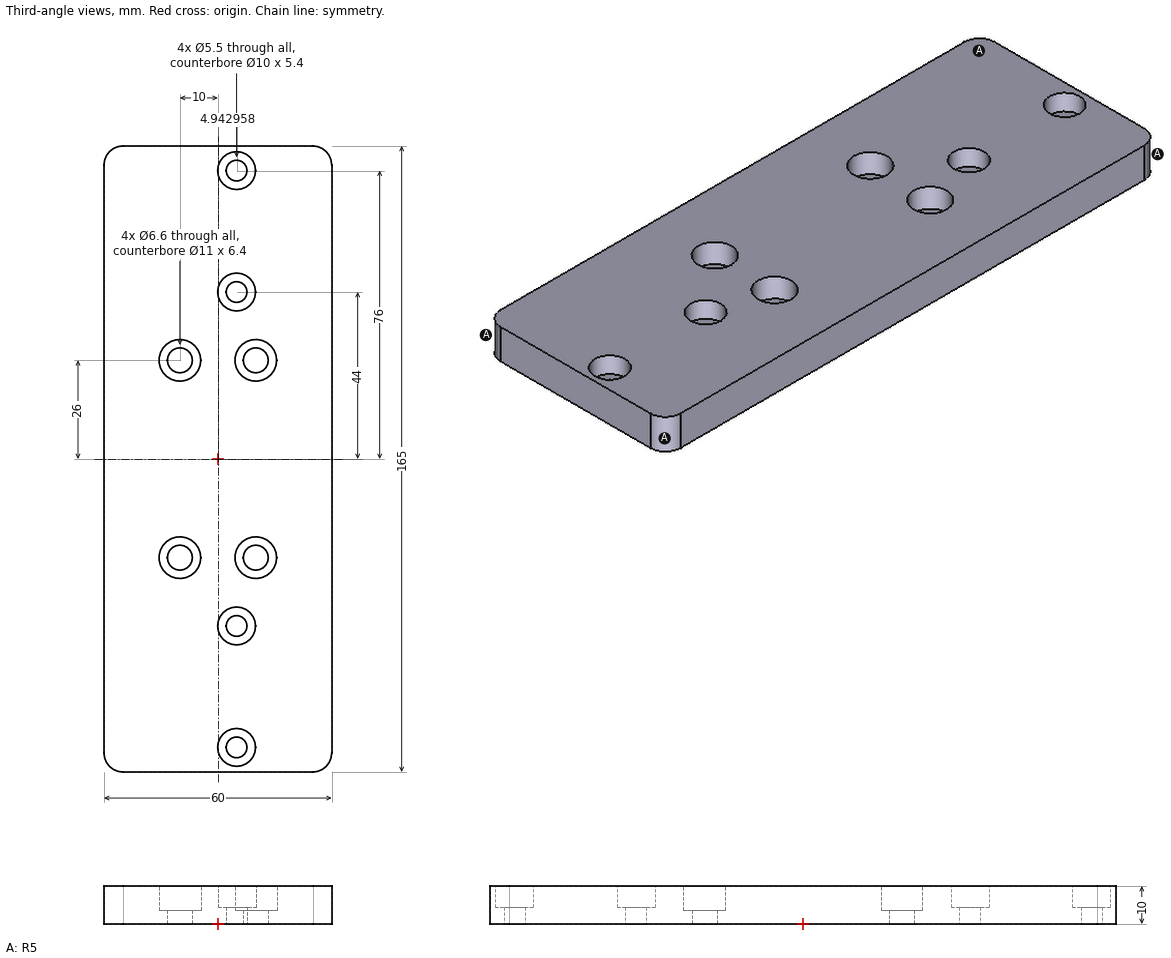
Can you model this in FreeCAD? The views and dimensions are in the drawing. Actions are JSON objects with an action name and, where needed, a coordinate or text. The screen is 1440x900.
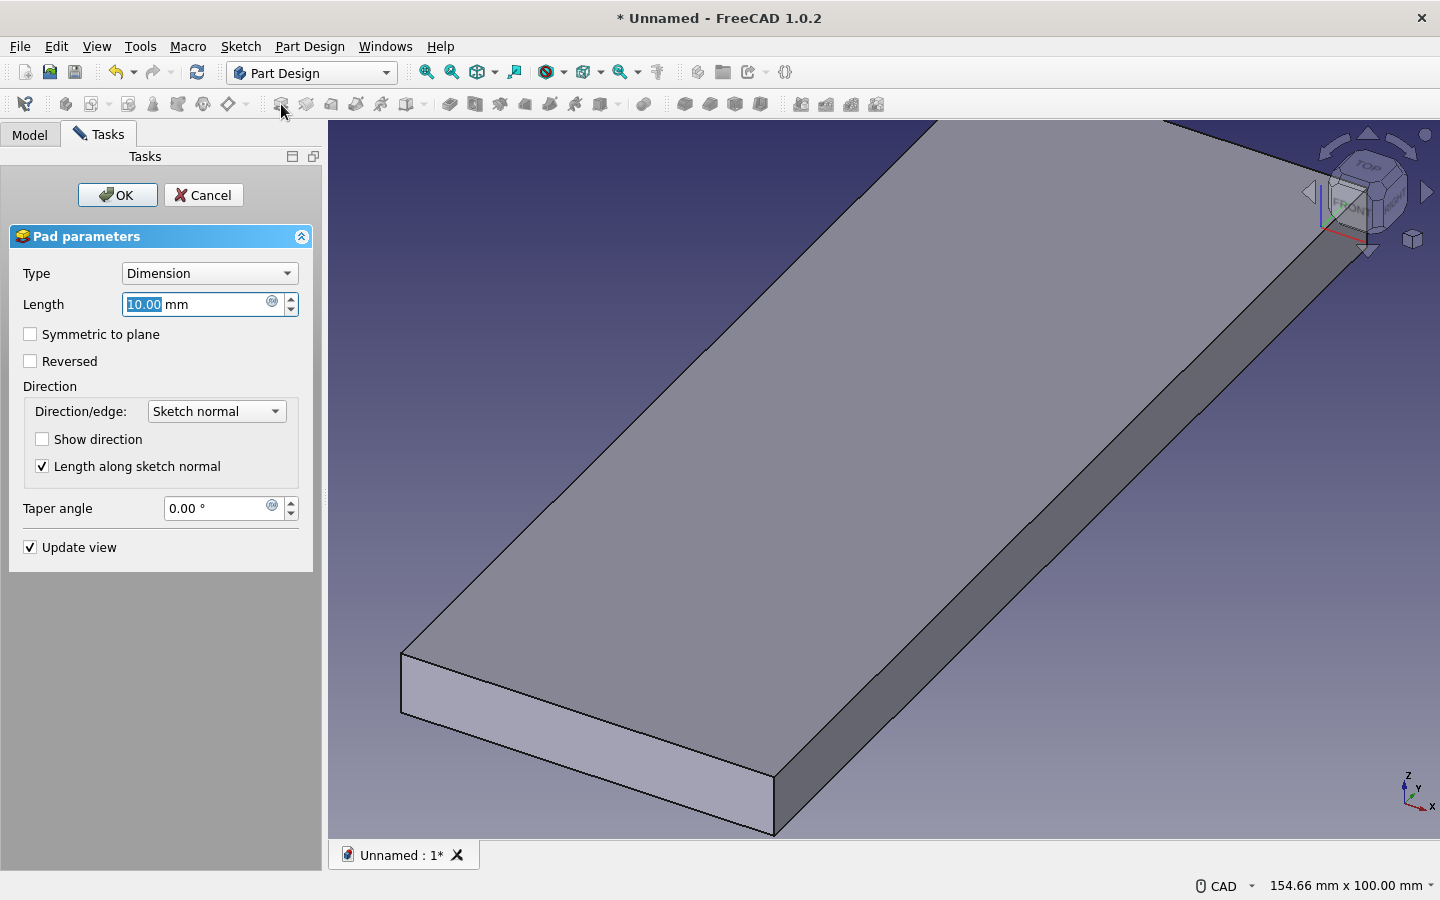
{"action": "type", "text": "10"}
{"action": "key", "text": "Tab"}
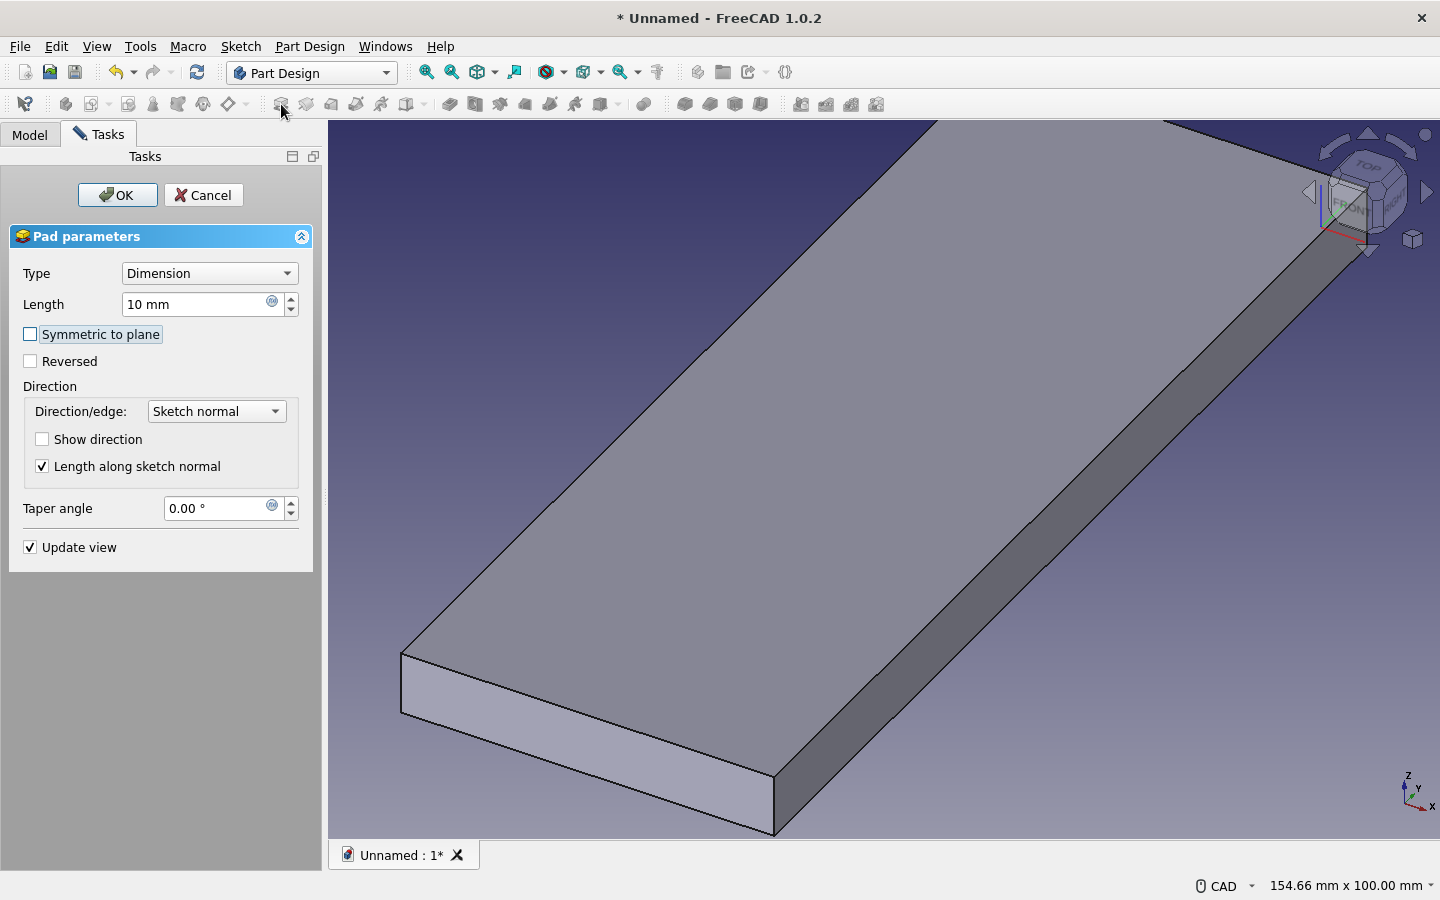
{"action": "left_click", "coordinate": [118, 195]}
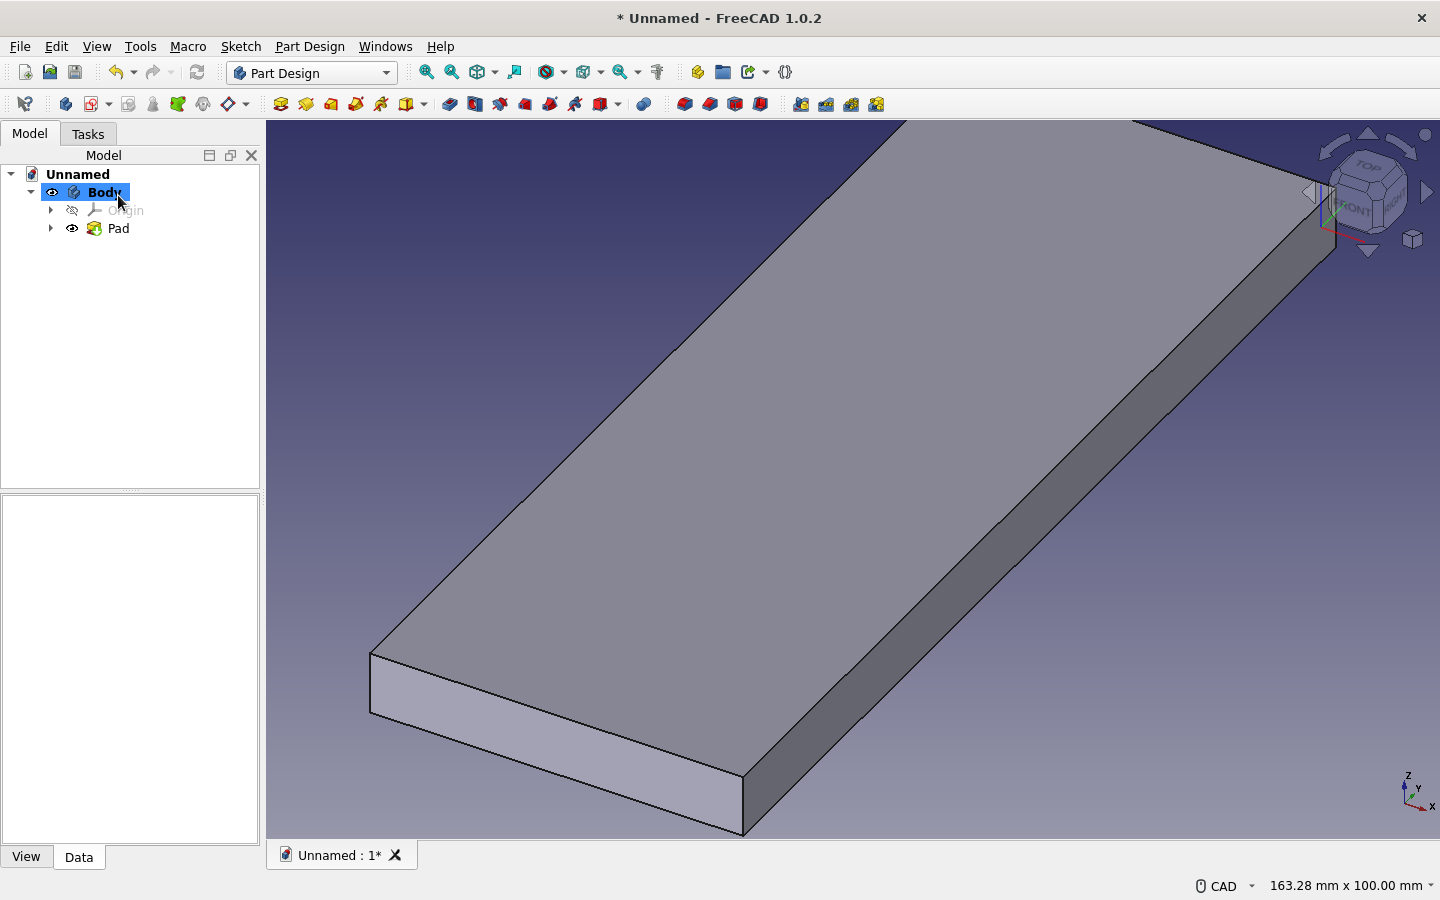
{"action": "left_click", "coordinate": [427, 72]}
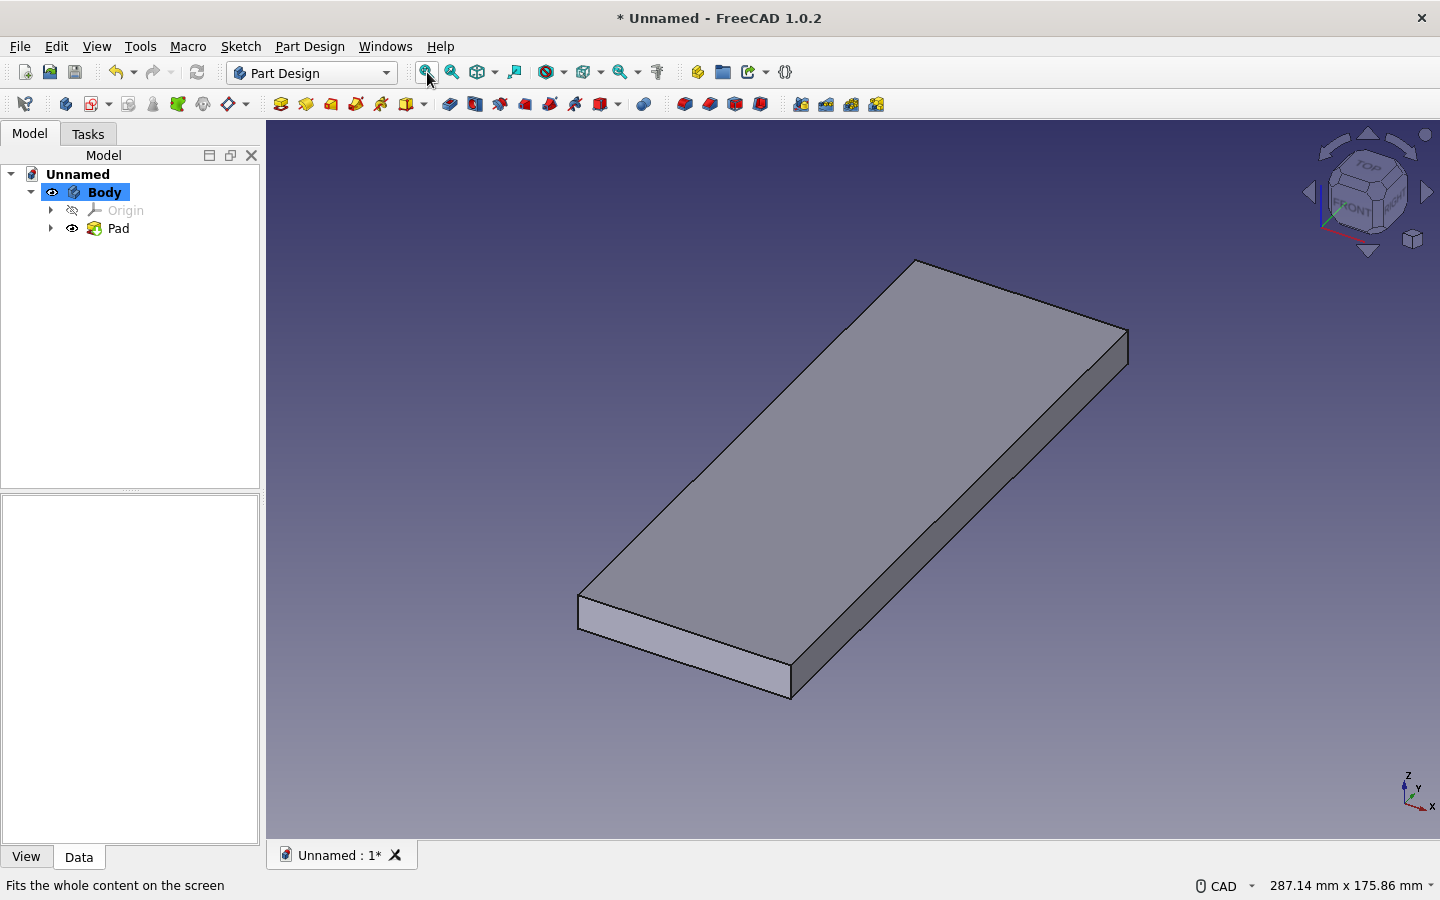
{"action": "left_click", "coordinate": [949, 366]}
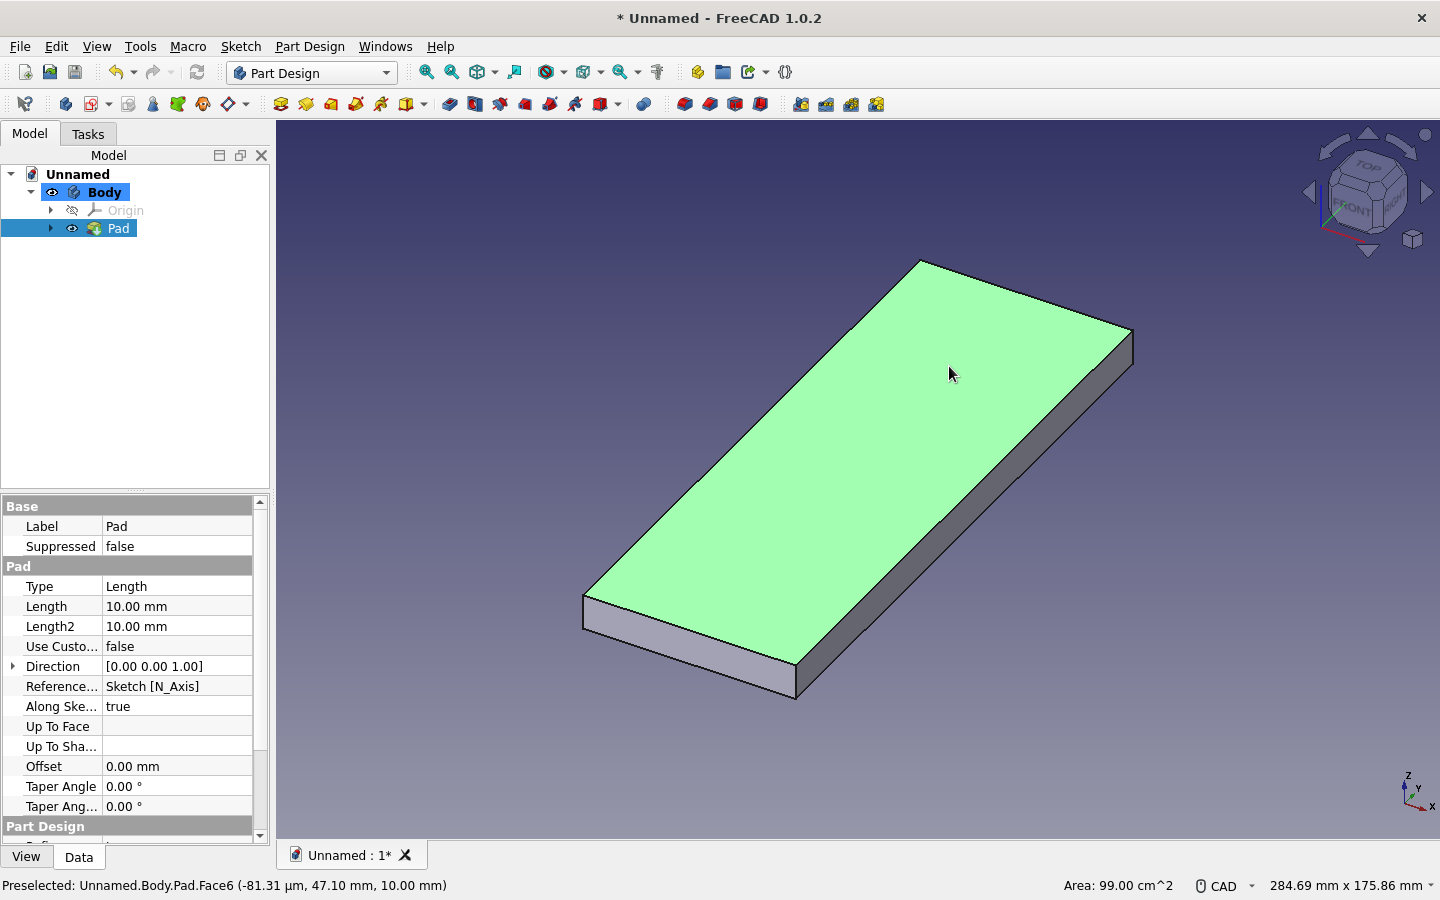
{"action": "left_click", "coordinate": [90, 104]}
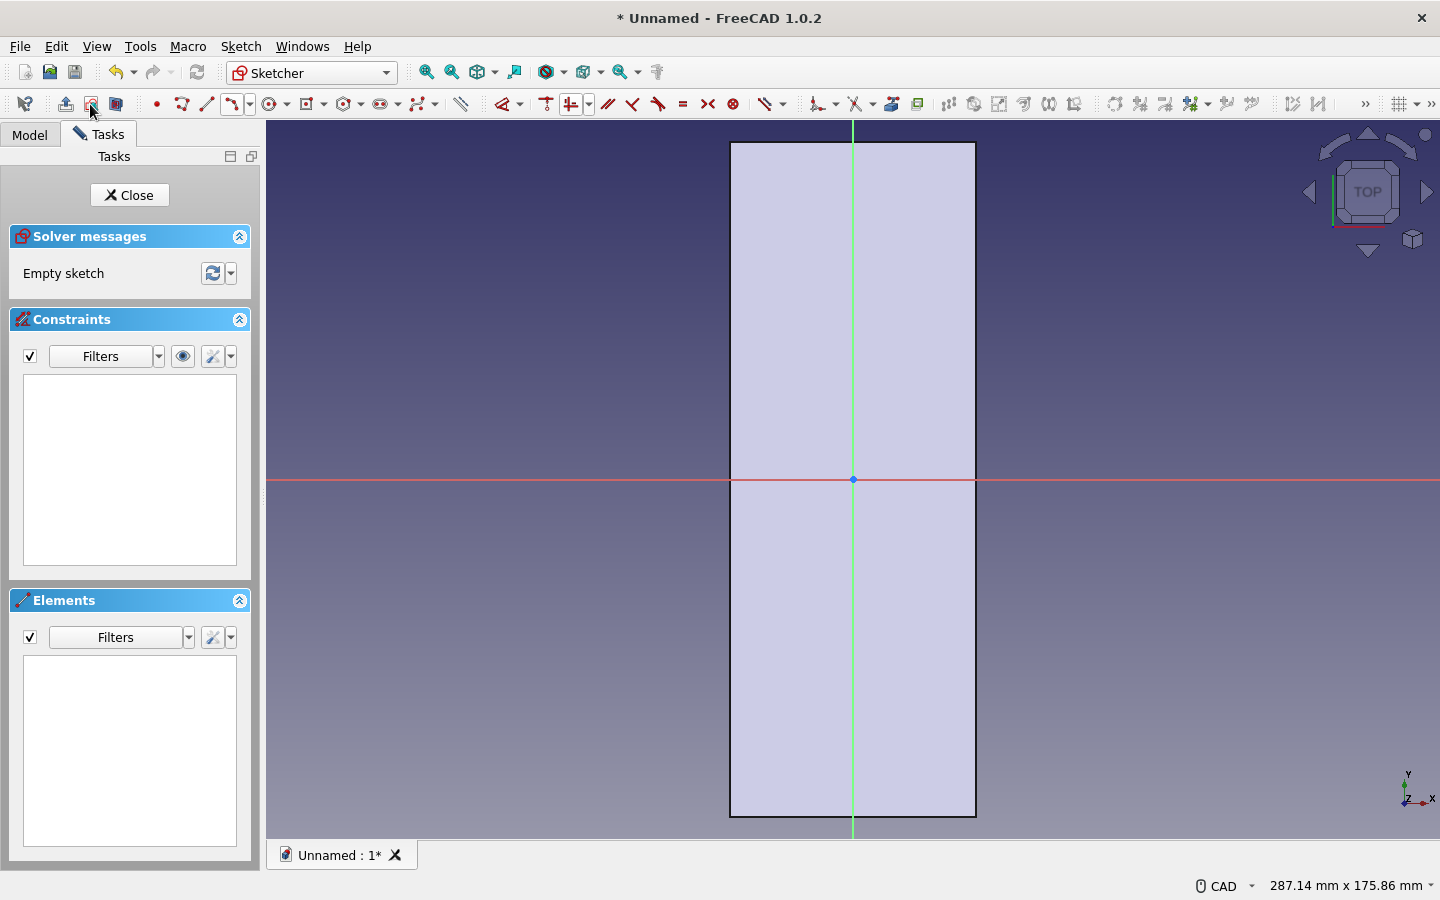
{"action": "scroll", "coordinate": [936, 480], "scroll_direction": "up", "scroll_amount": 3}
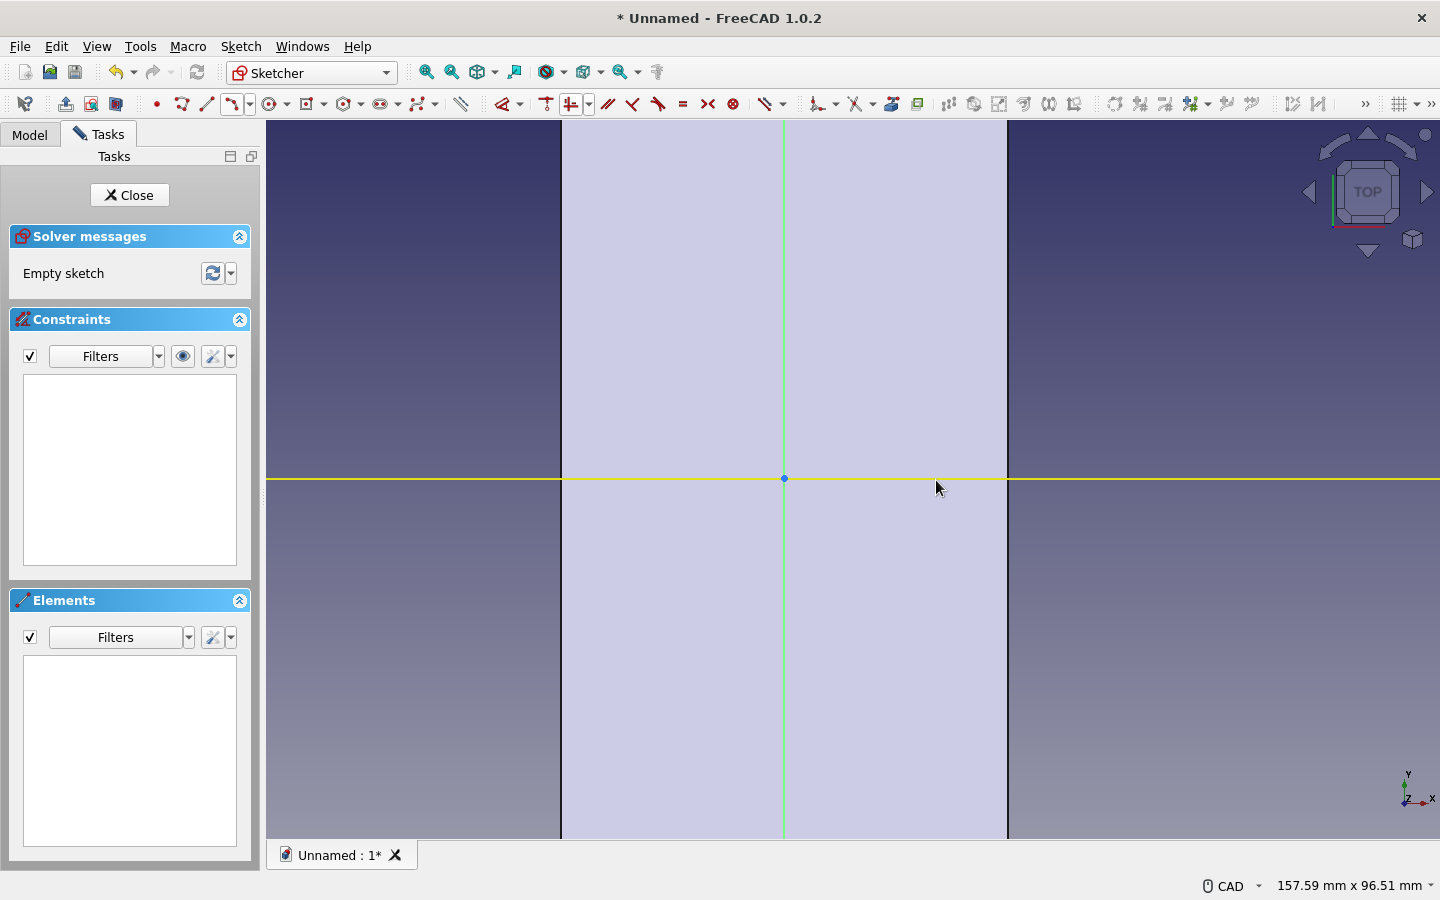
{"action": "left_click", "coordinate": [268, 104]}